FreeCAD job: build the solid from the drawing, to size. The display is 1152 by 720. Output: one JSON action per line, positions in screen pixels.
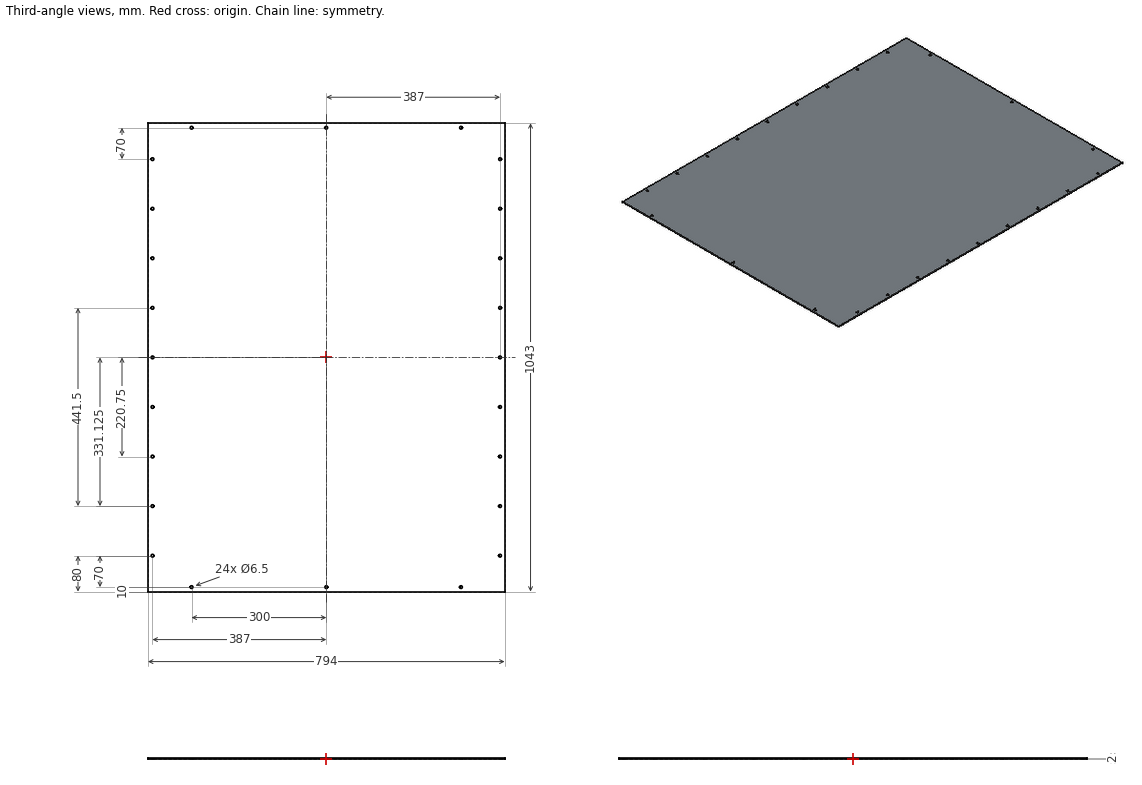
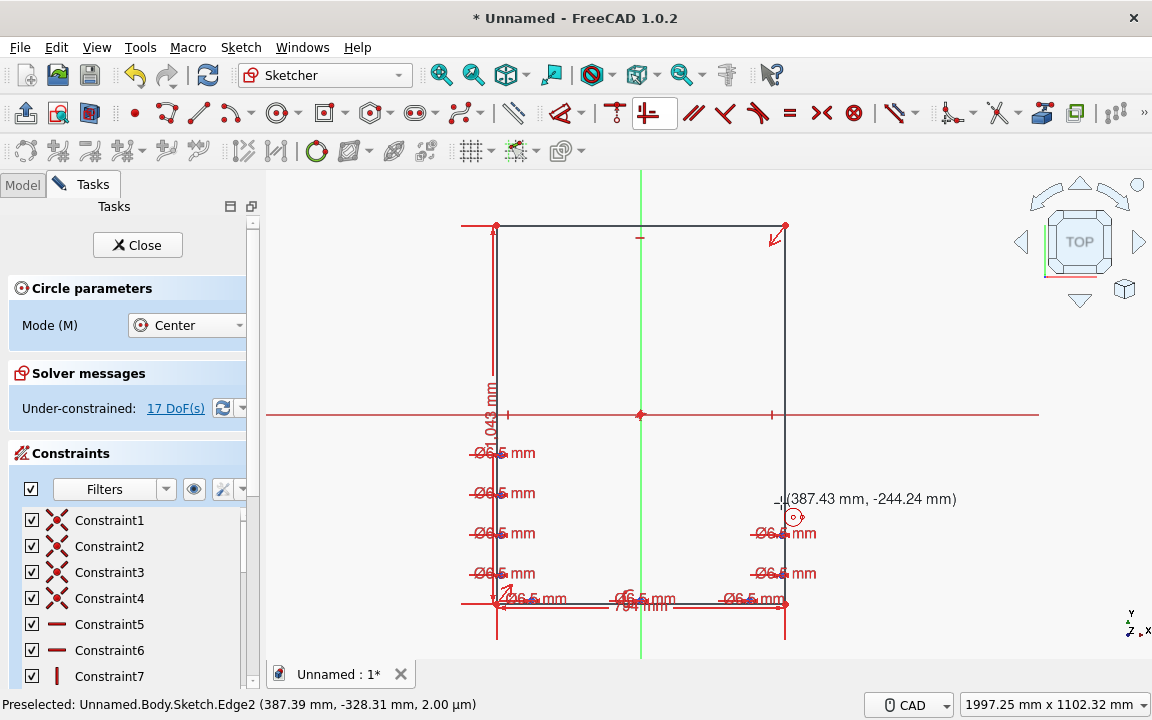
{"action": "scroll", "coordinate": [781, 495], "scroll_direction": "up", "scroll_amount": 8}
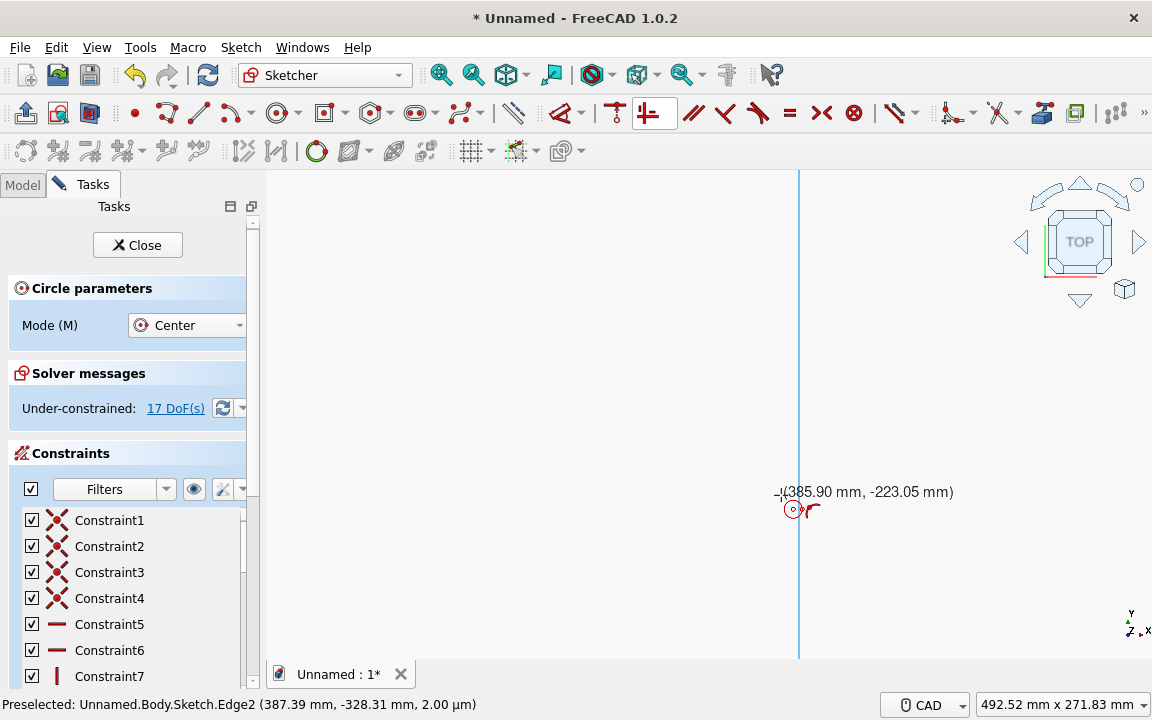
{"action": "left_click", "coordinate": [781, 493]}
{"action": "mouse_move", "coordinate": [777, 489]}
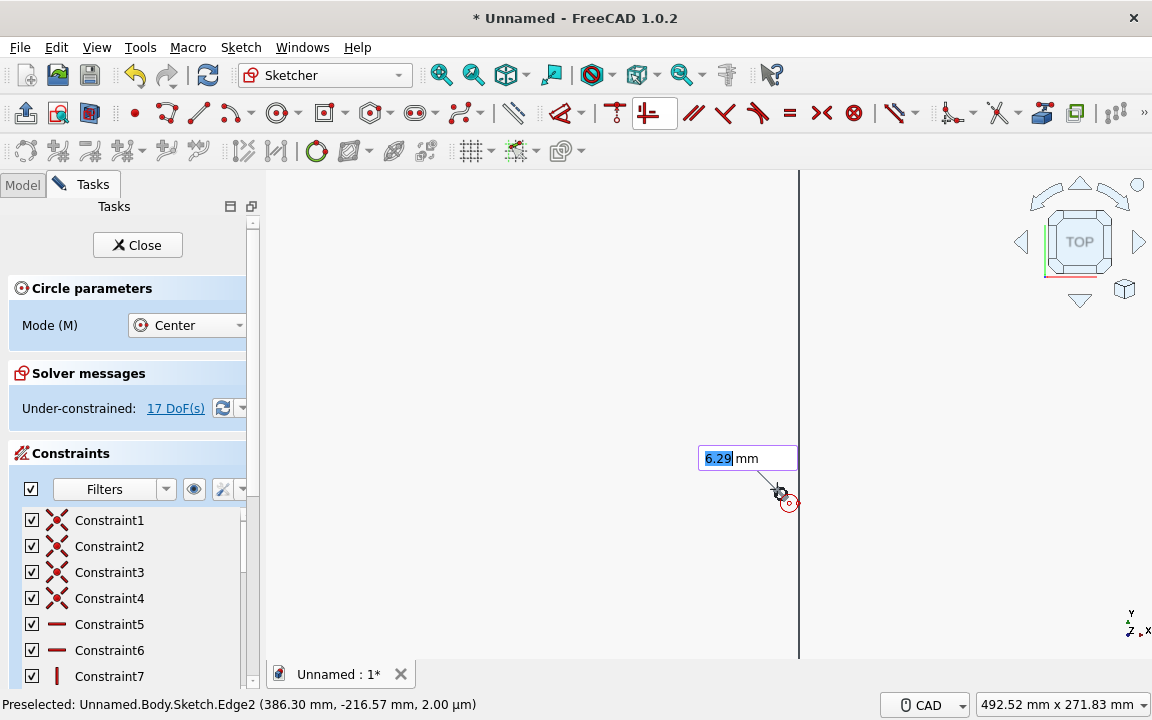
{"action": "type", "text": "6.5"}
{"action": "key", "text": "Return"}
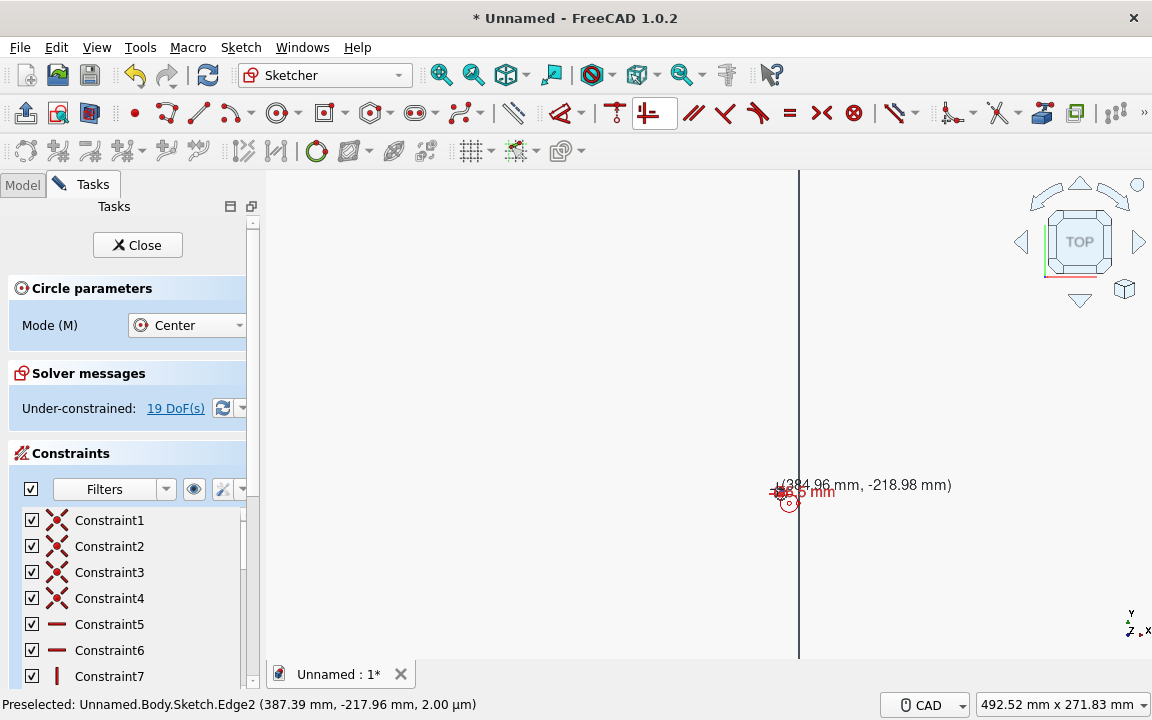
{"action": "scroll", "coordinate": [781, 295], "scroll_direction": "up", "scroll_amount": 7}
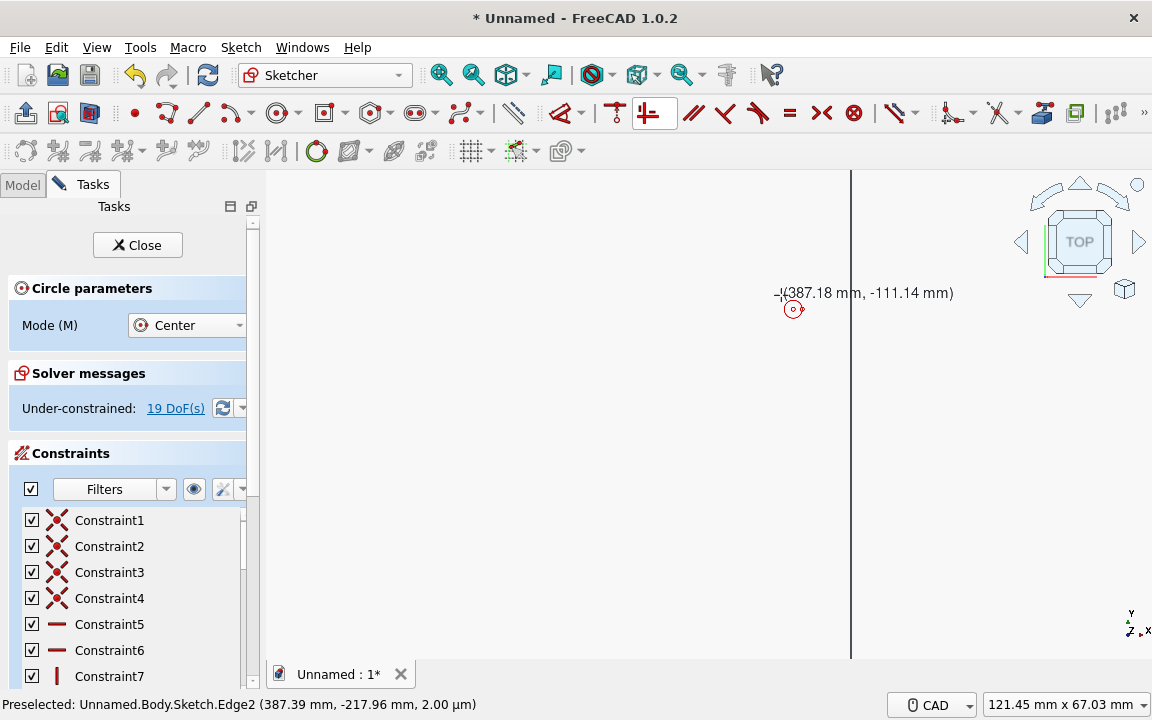
{"action": "scroll", "coordinate": [781, 463], "scroll_direction": "down", "scroll_amount": 15}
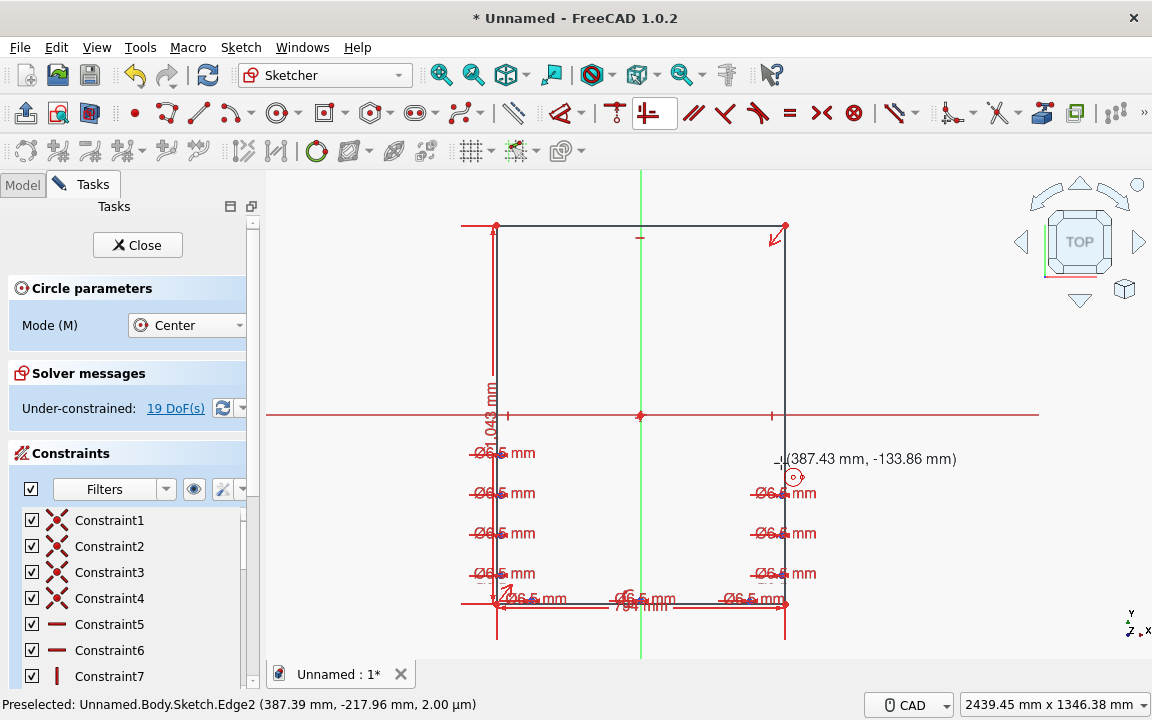
{"action": "scroll", "coordinate": [781, 455], "scroll_direction": "up", "scroll_amount": 8}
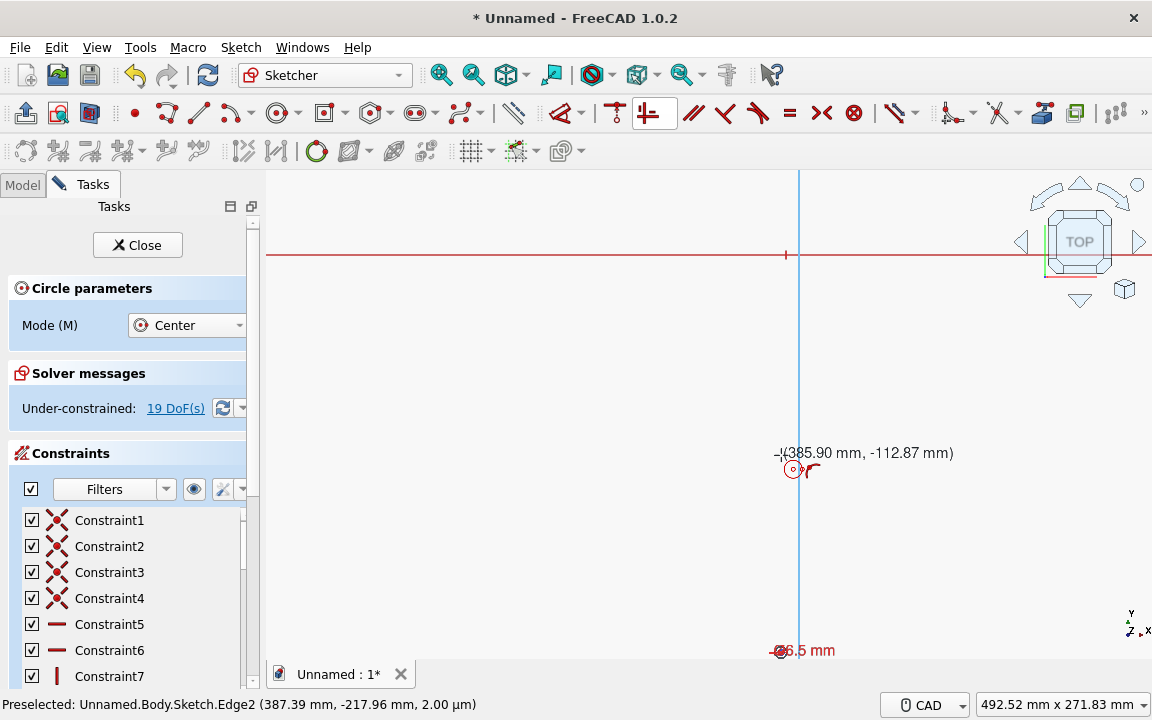
{"action": "left_click", "coordinate": [781, 453]}
{"action": "mouse_move", "coordinate": [777, 449]}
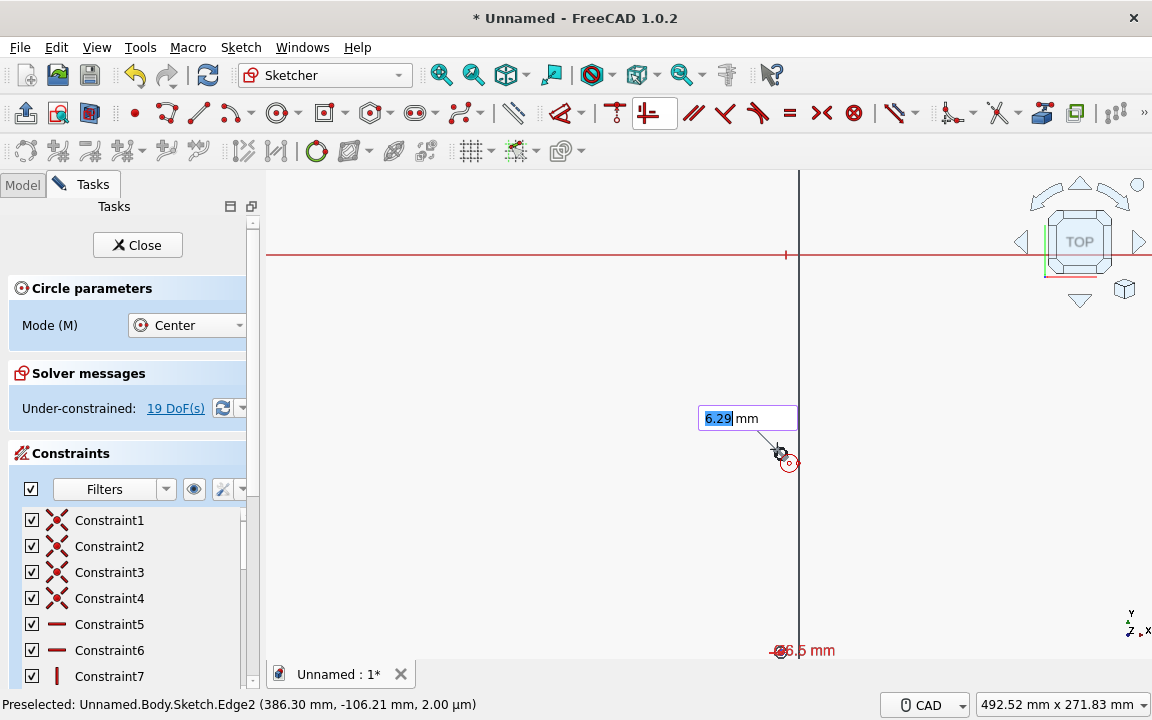
{"action": "type", "text": "6.5"}
{"action": "key", "text": "Return"}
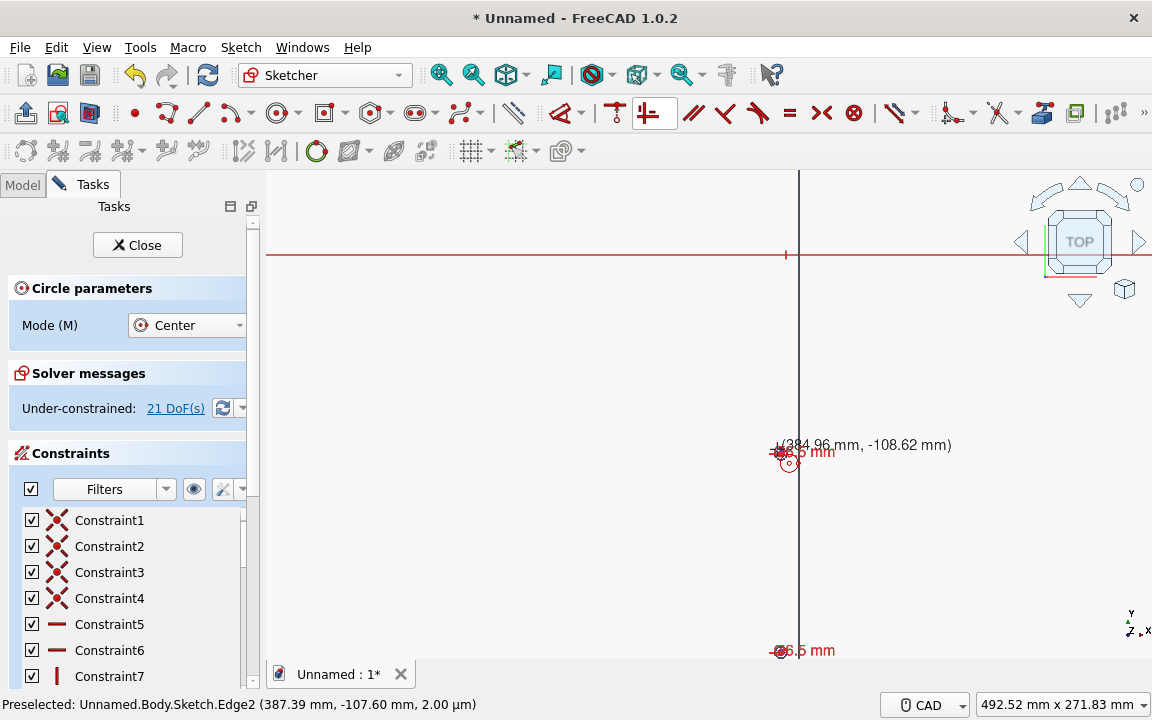
{"action": "scroll", "coordinate": [751, 446], "scroll_direction": "down", "scroll_amount": 9}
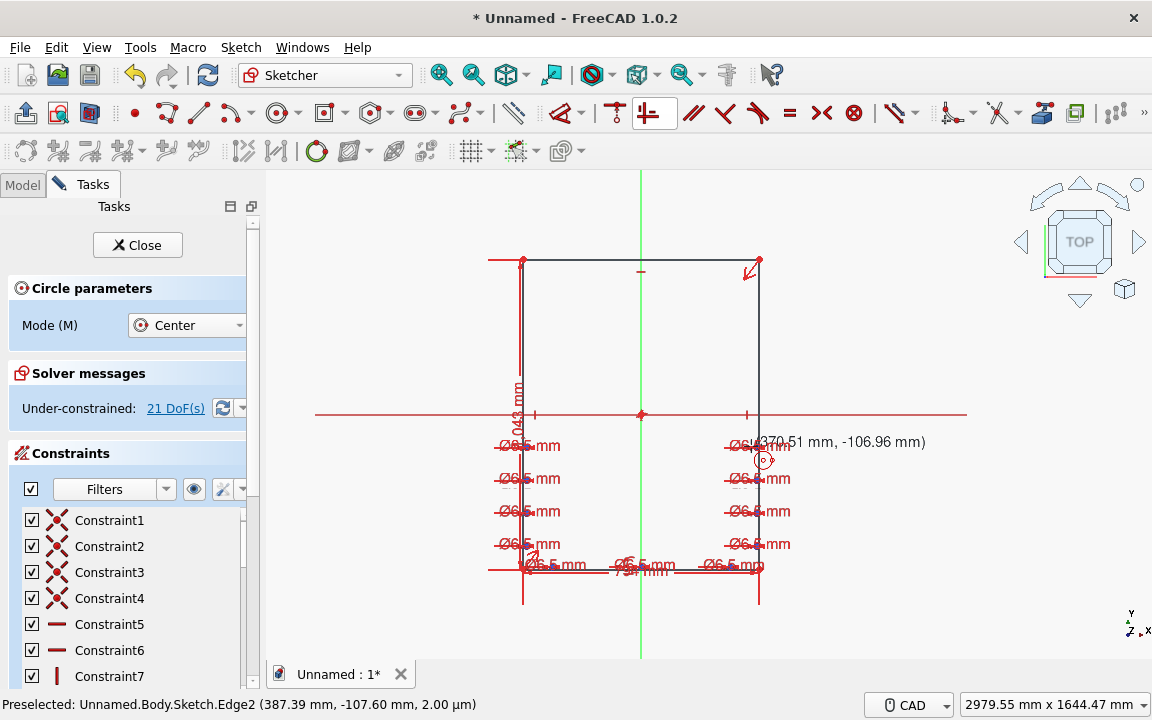
{"action": "scroll", "coordinate": [526, 415], "scroll_direction": "up", "scroll_amount": 16}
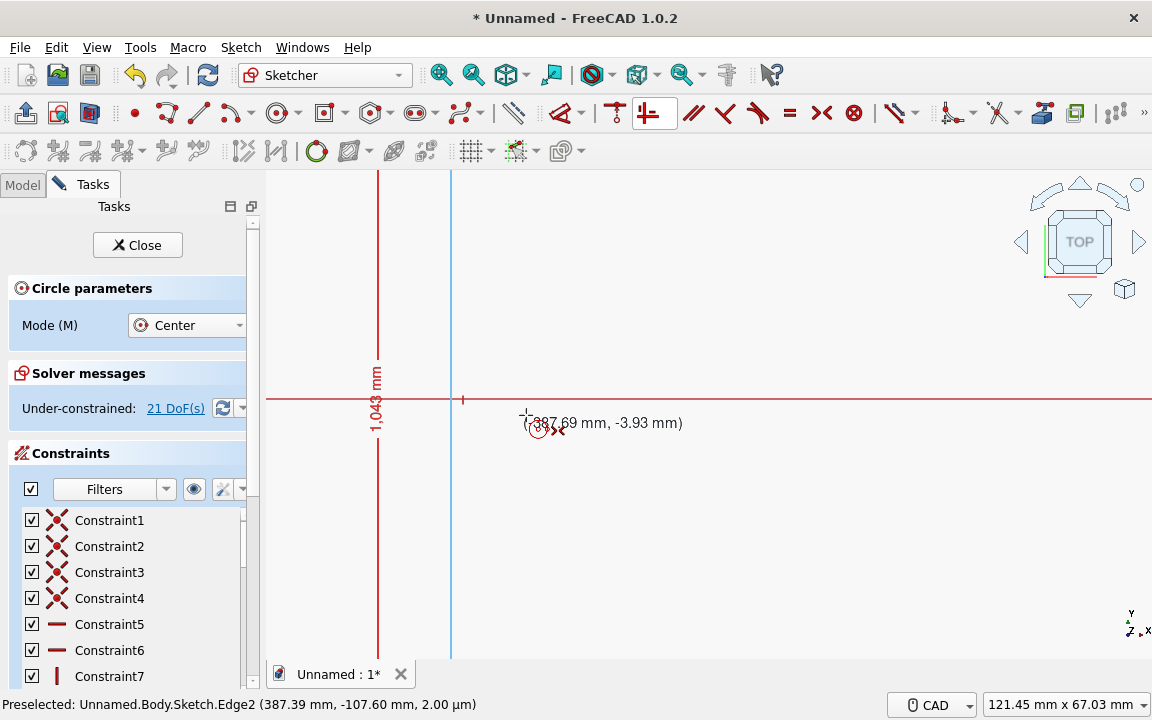
{"action": "scroll", "coordinate": [499, 415], "scroll_direction": "down", "scroll_amount": 15}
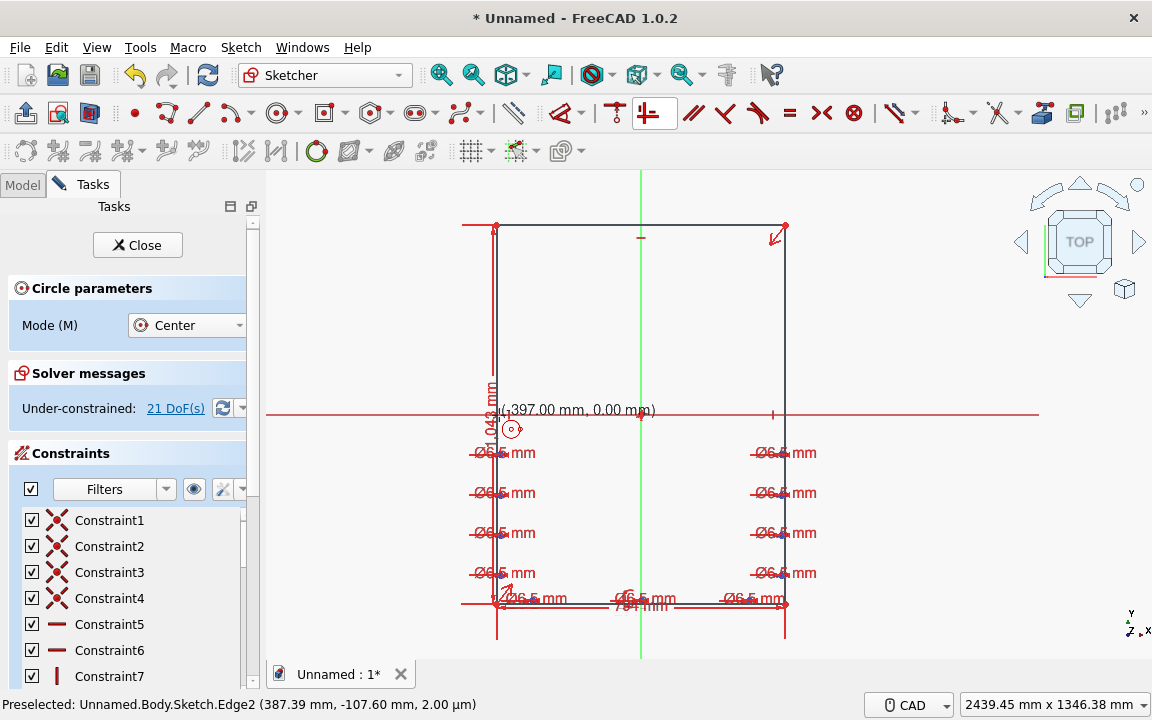
{"action": "scroll", "coordinate": [501, 415], "scroll_direction": "up", "scroll_amount": 8}